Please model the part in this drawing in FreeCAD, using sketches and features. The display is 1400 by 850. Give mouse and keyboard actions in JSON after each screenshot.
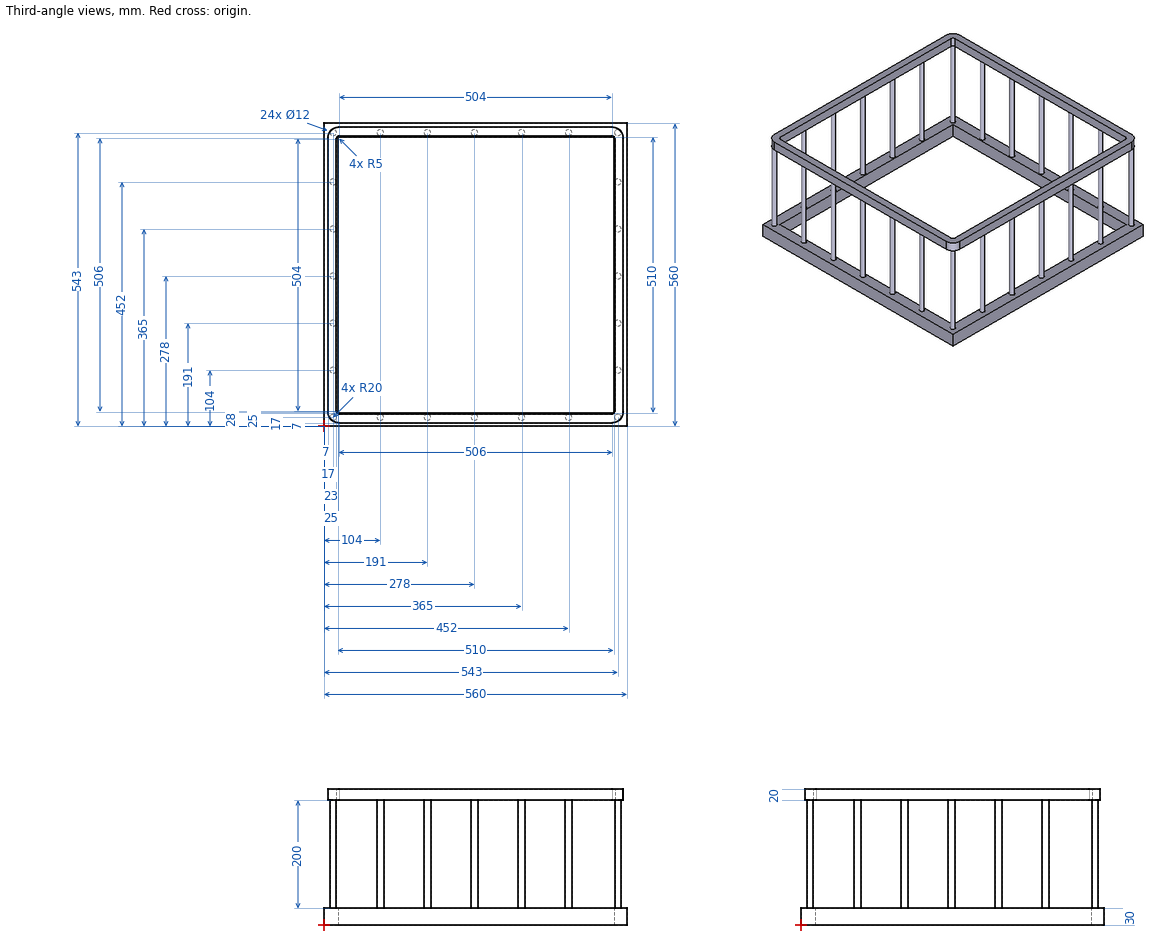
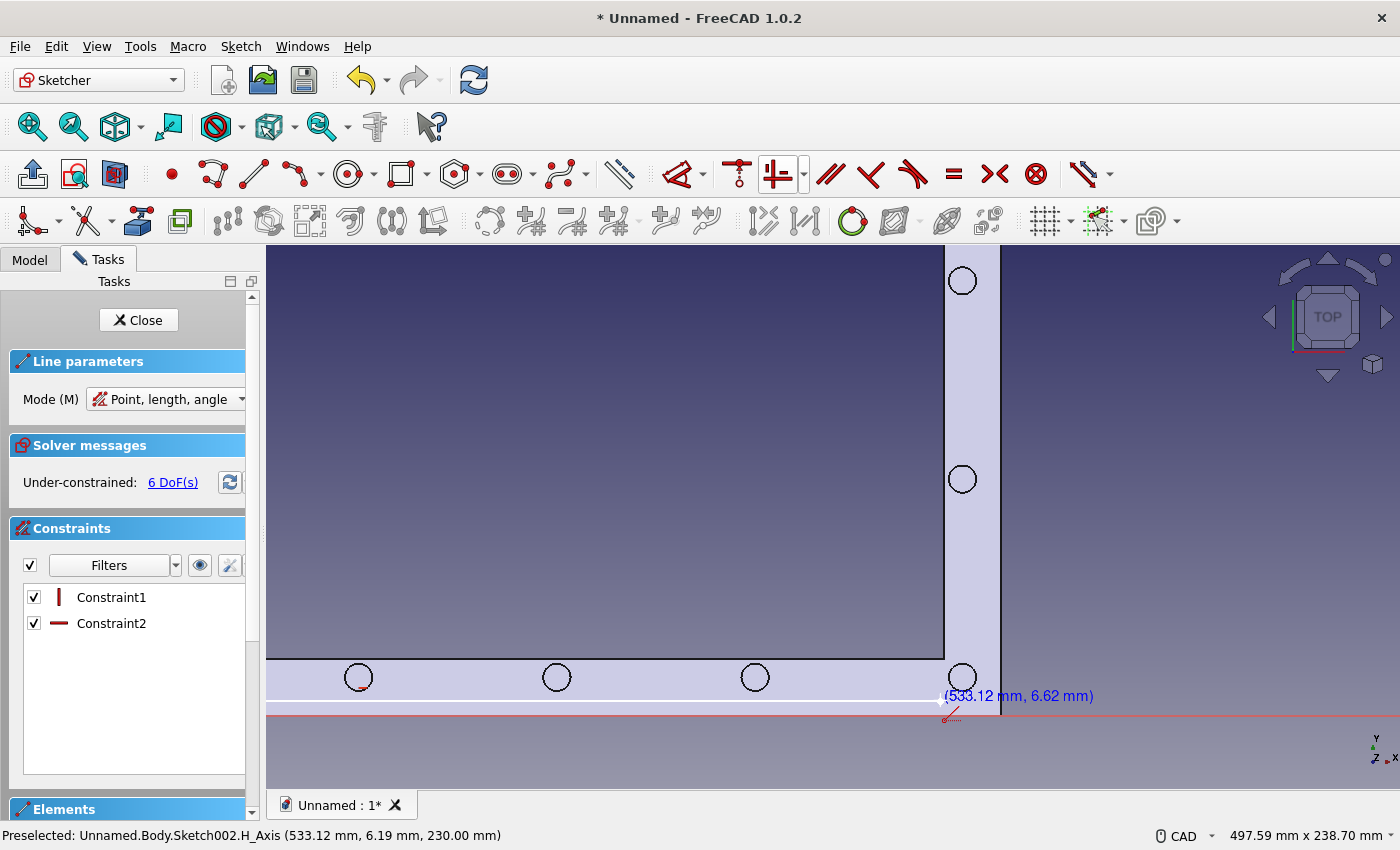
{"action": "left_click", "coordinate": [985, 655]}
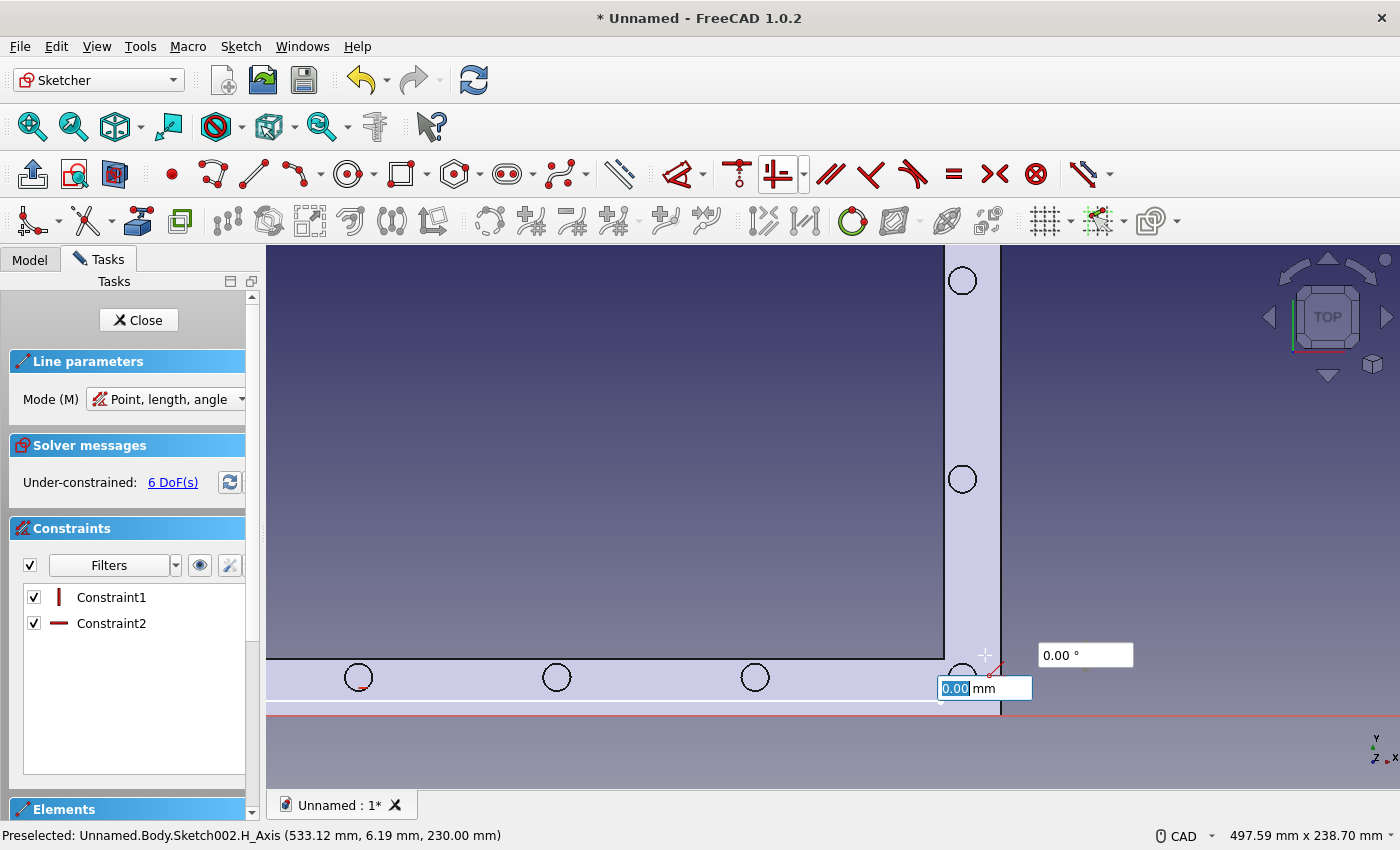
{"action": "scroll", "coordinate": [941, 703], "scroll_direction": "down", "scroll_amount": 6}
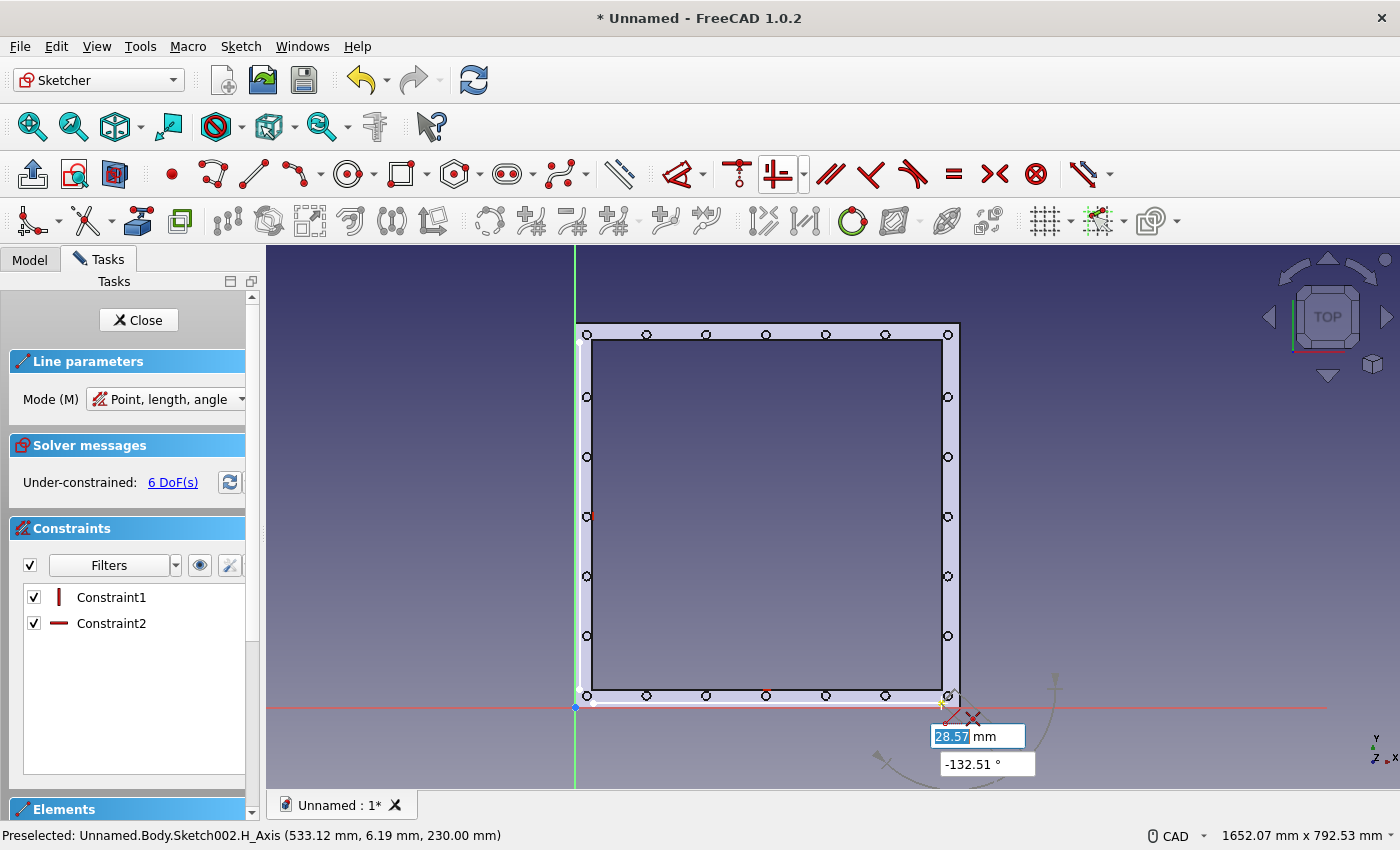
{"action": "left_click", "coordinate": [955, 342]}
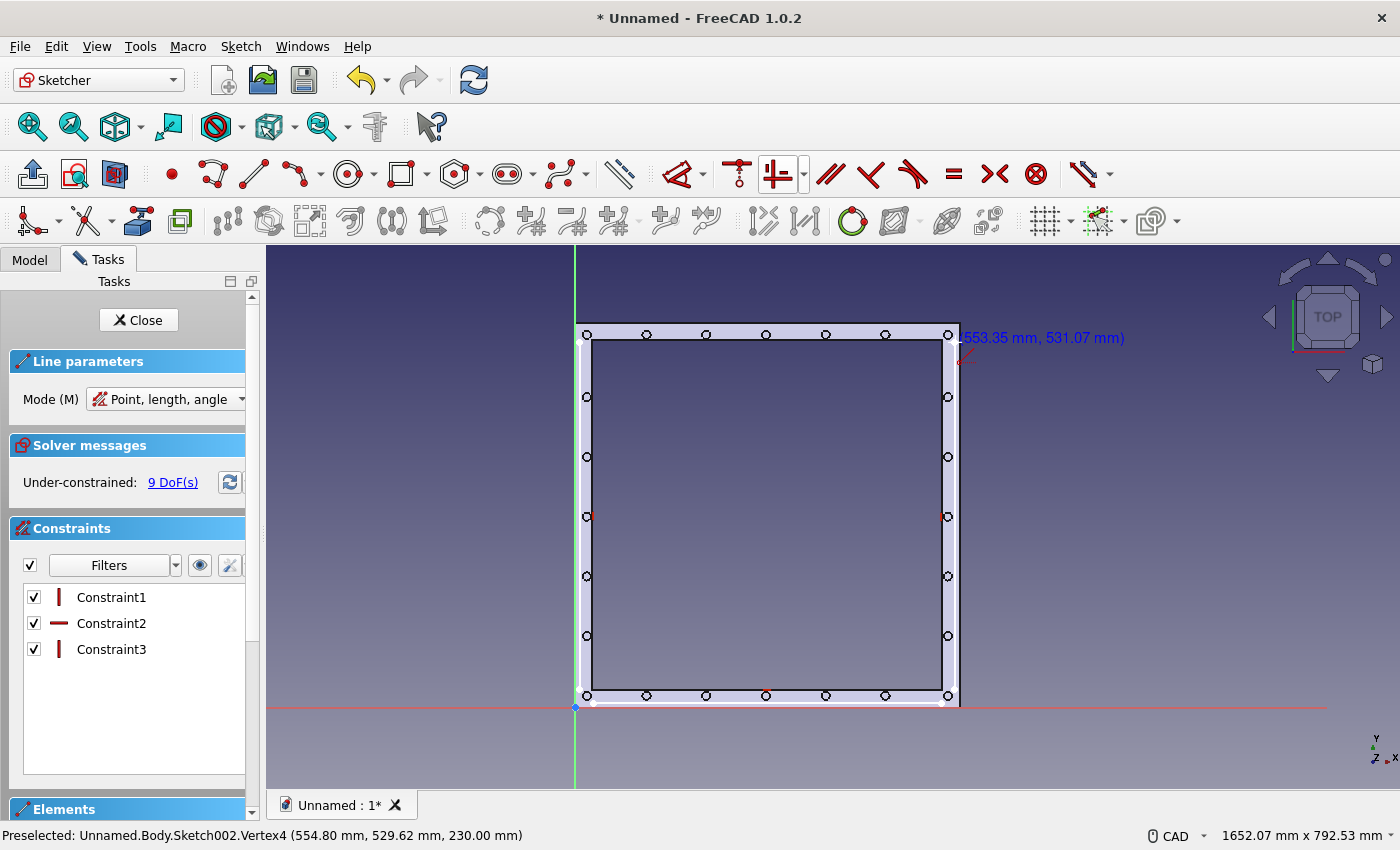
{"action": "left_click", "coordinate": [941, 328]}
{"action": "left_click", "coordinate": [594, 328]}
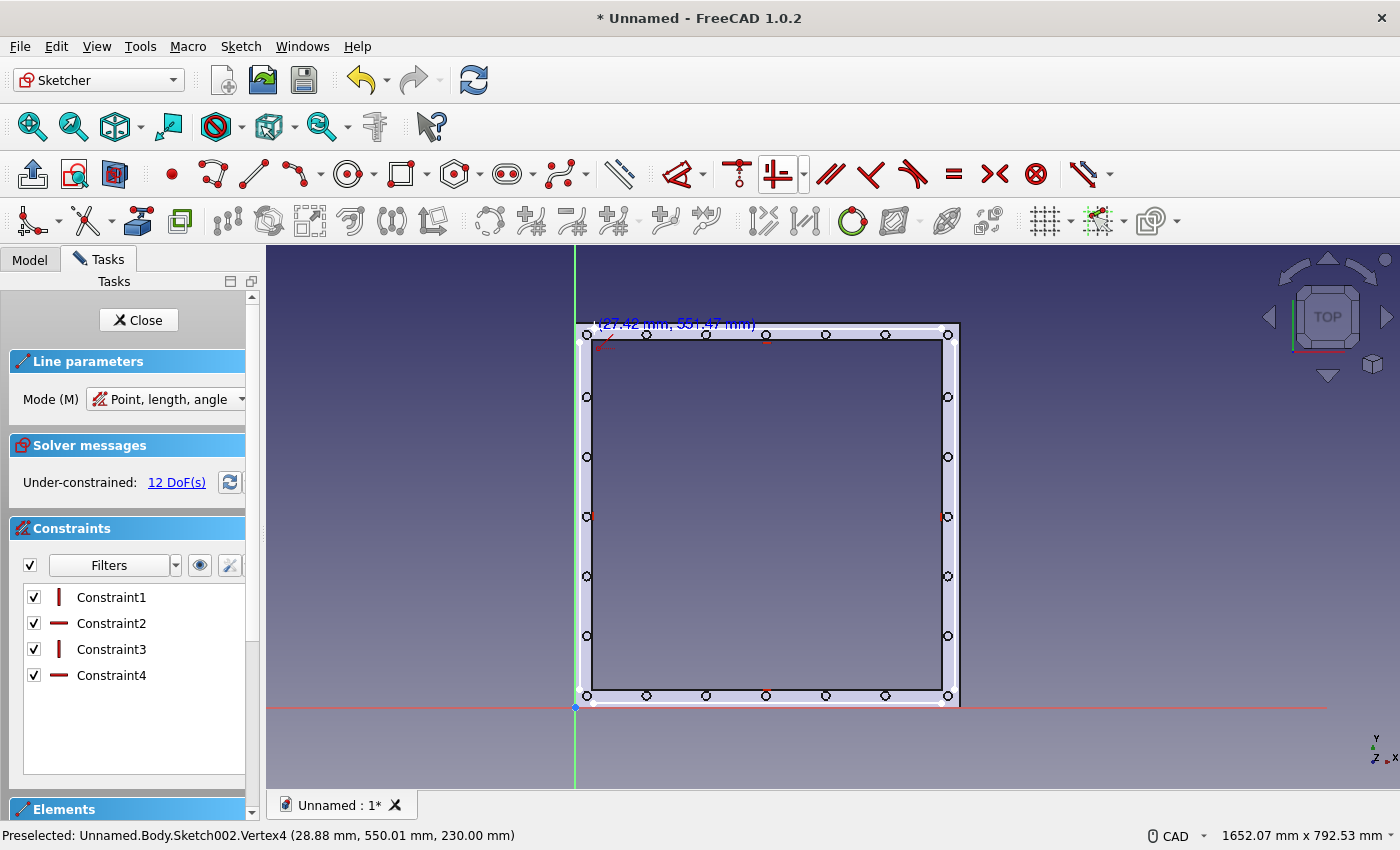
{"action": "left_click", "coordinate": [294, 174]}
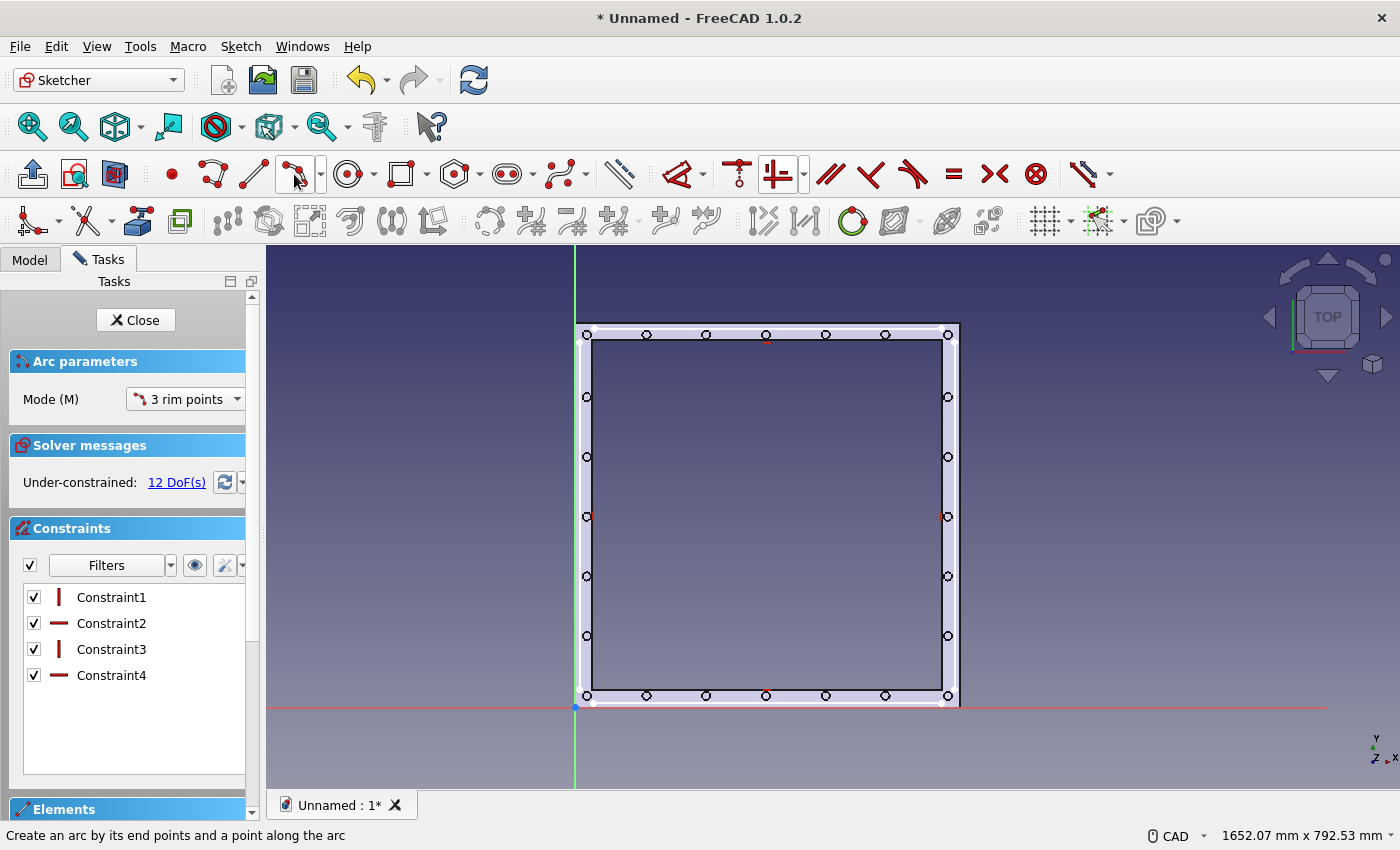
{"action": "scroll", "coordinate": [580, 689], "scroll_direction": "up", "scroll_amount": 6}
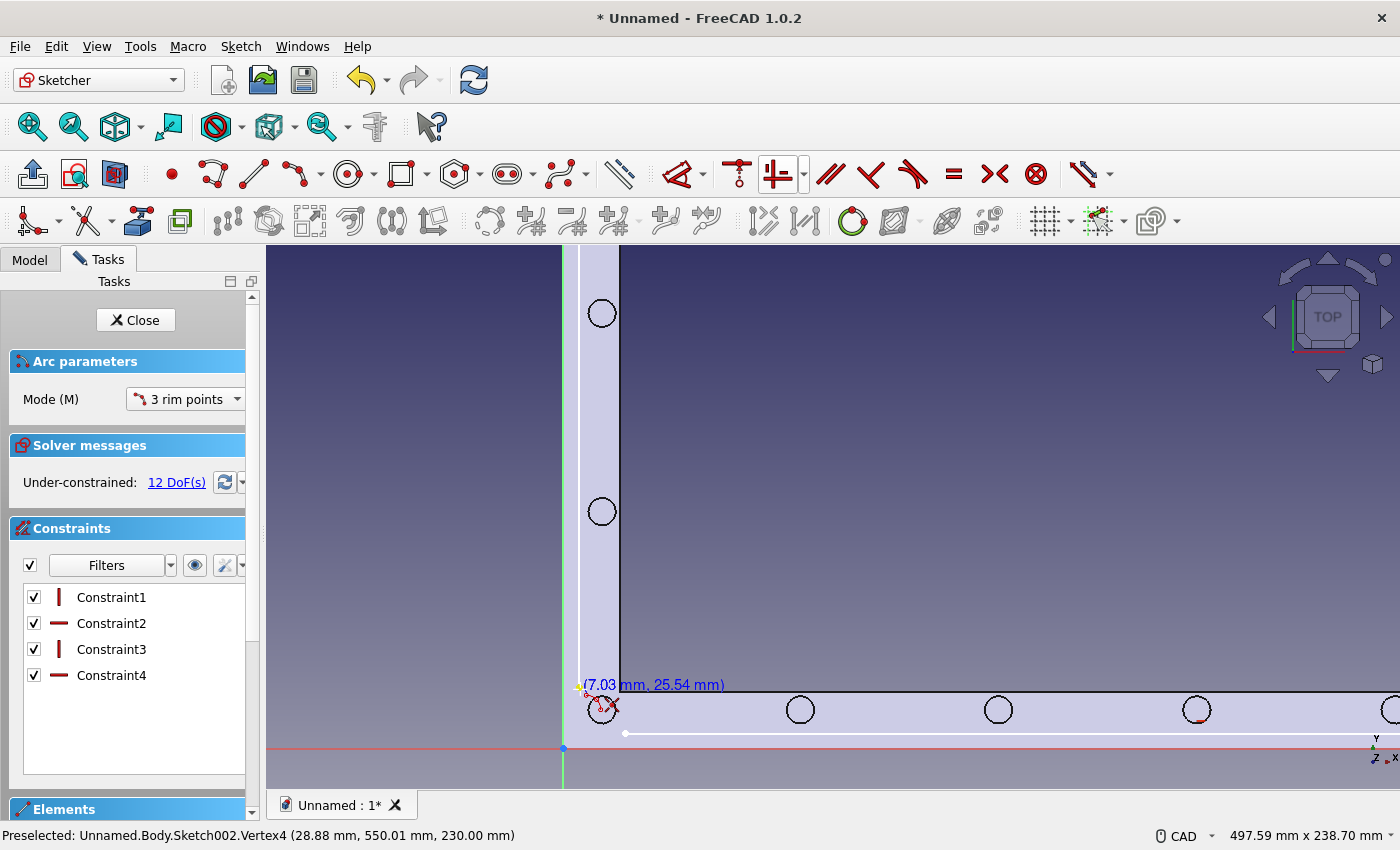
{"action": "left_click", "coordinate": [579, 688]}
{"action": "left_click", "coordinate": [625, 734]}
{"action": "left_click", "coordinate": [593, 719]}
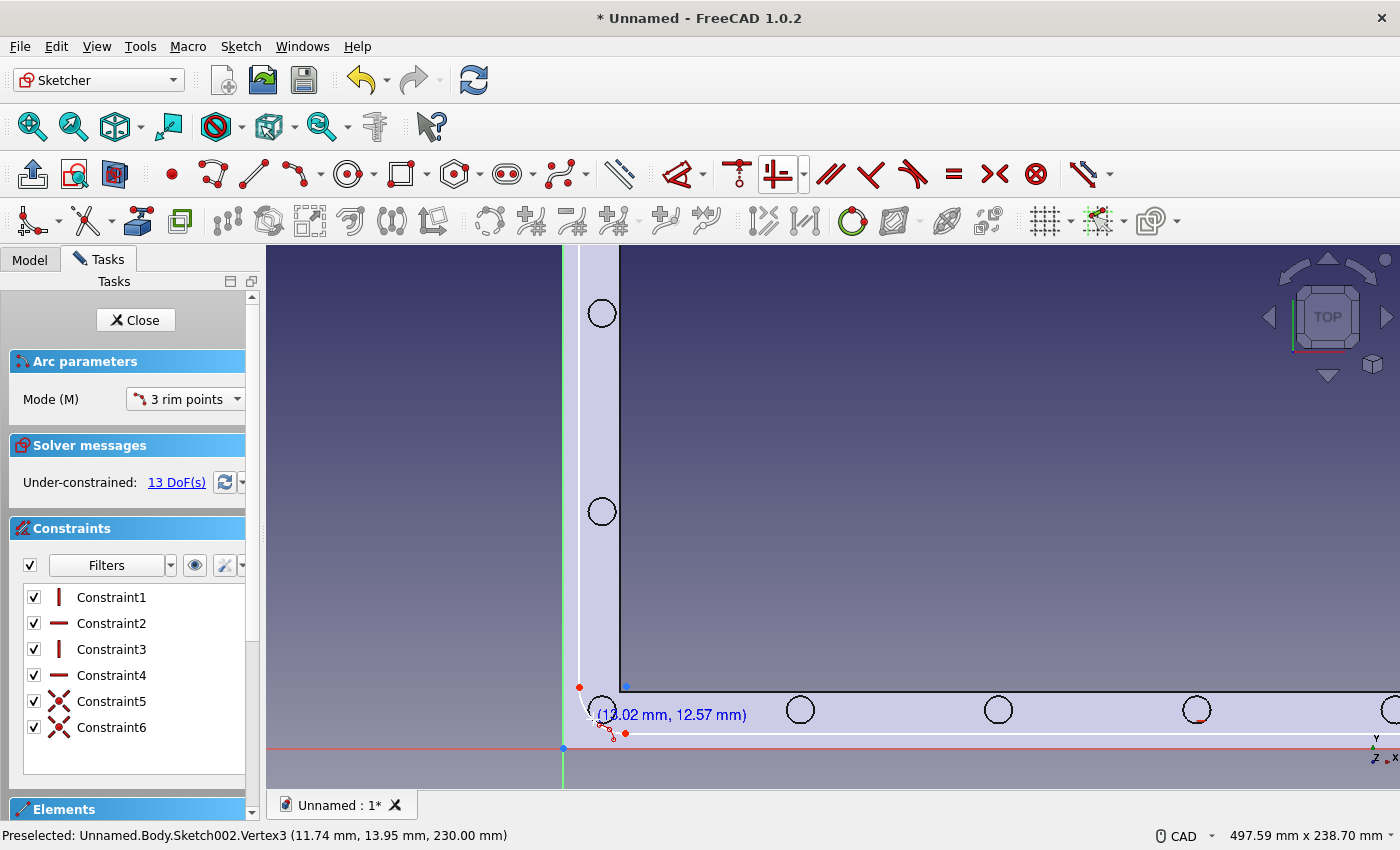
{"action": "scroll", "coordinate": [580, 689], "scroll_direction": "down", "scroll_amount": 6}